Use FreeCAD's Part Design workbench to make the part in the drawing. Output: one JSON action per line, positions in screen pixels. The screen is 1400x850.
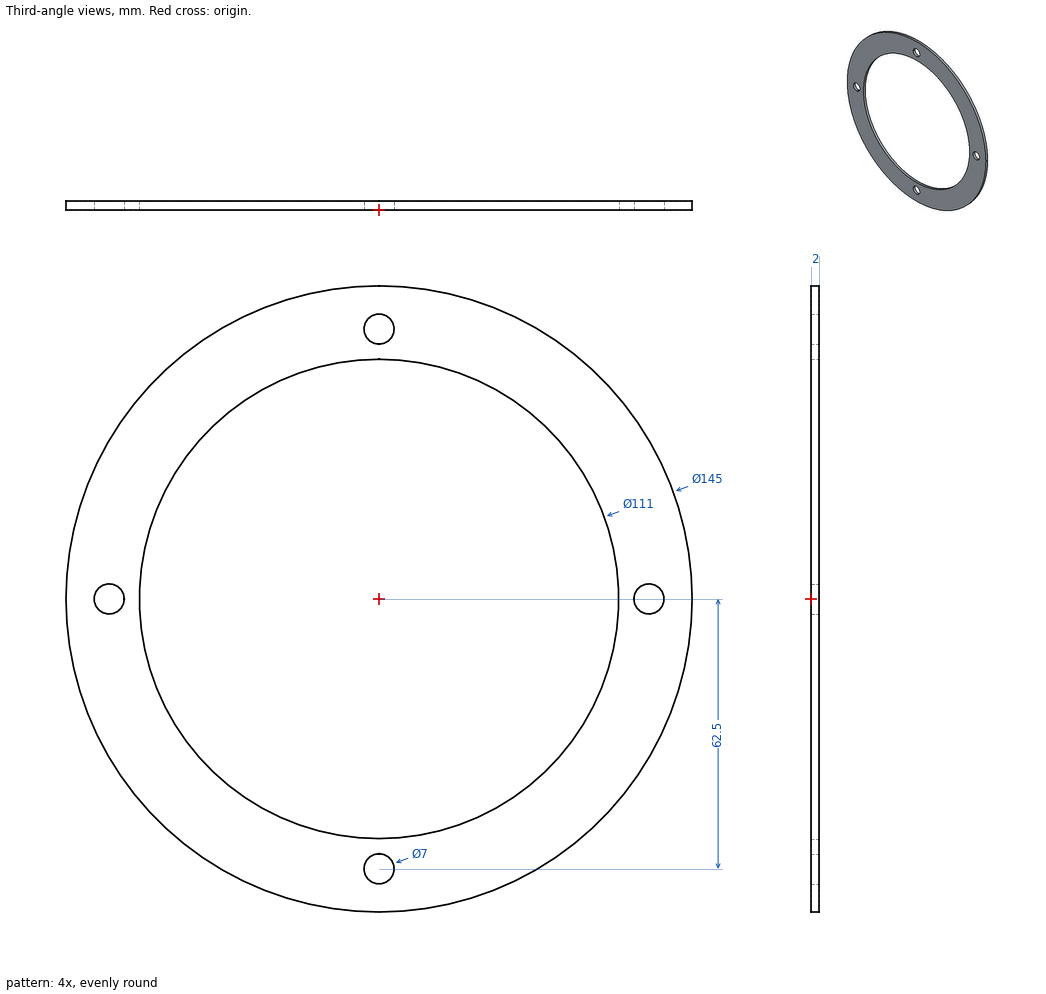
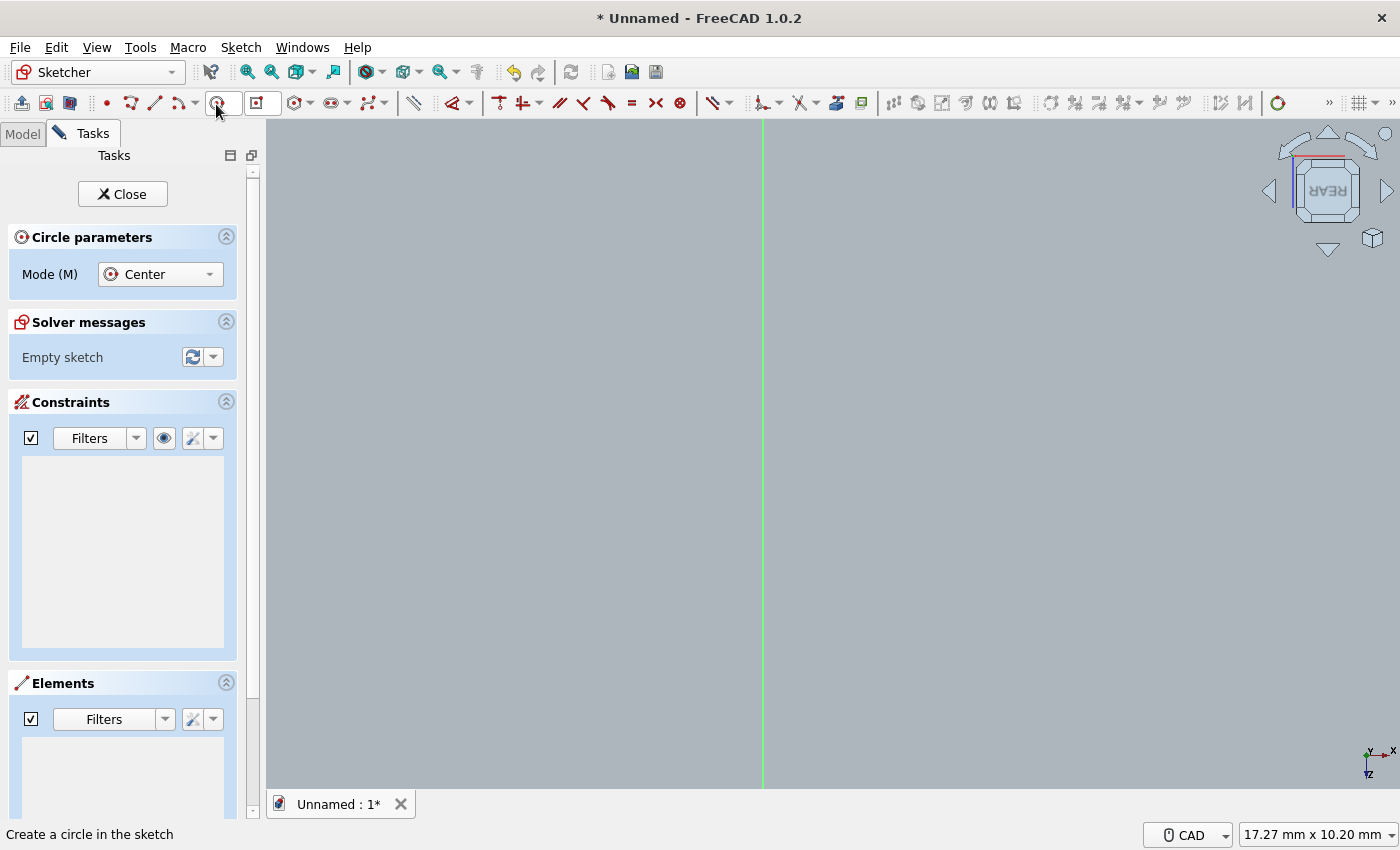
{"action": "left_click", "coordinate": [763, 451]}
{"action": "left_click", "coordinate": [925, 288]}
{"action": "key", "text": "Escape"}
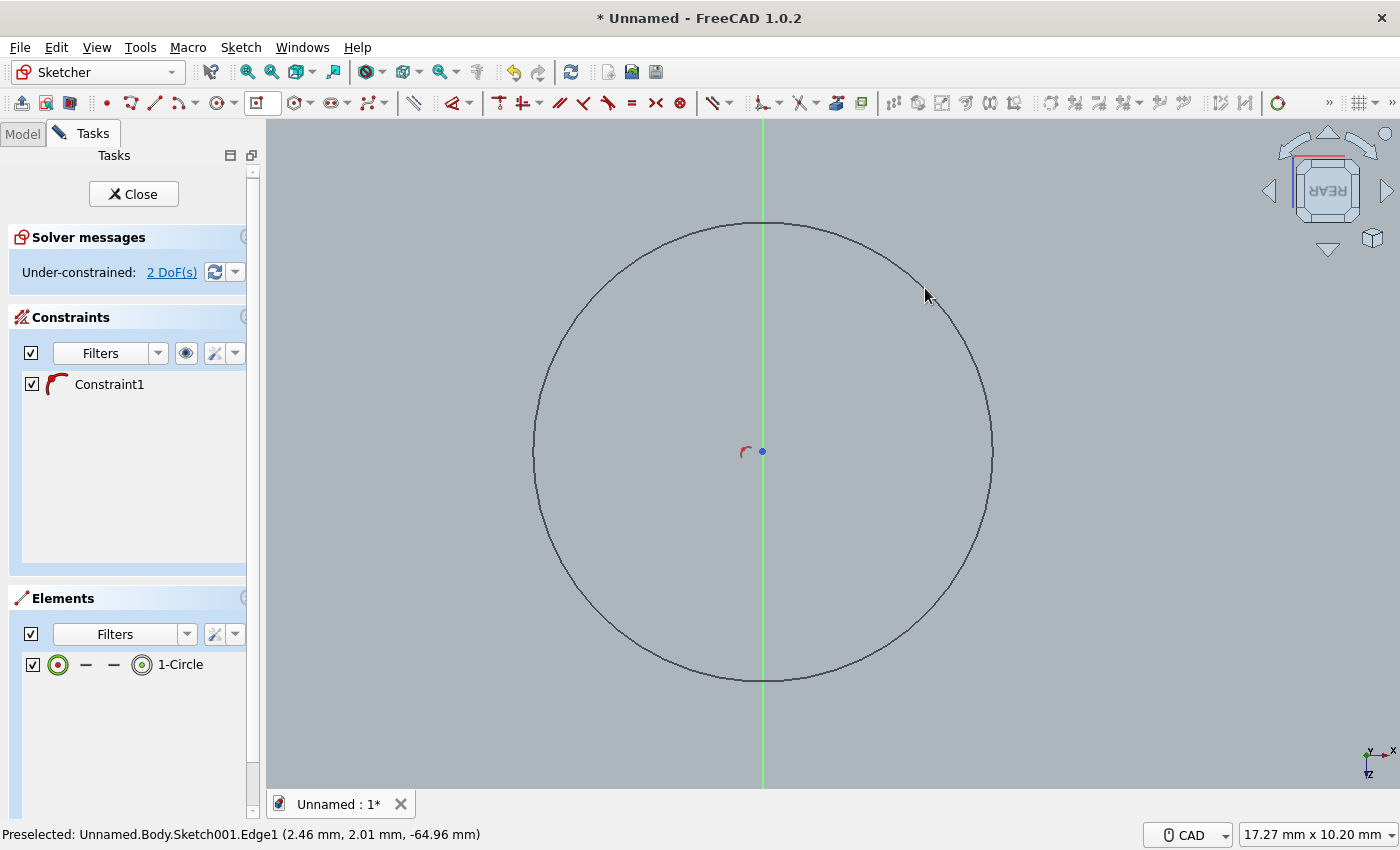
{"action": "left_click", "coordinate": [452, 104]}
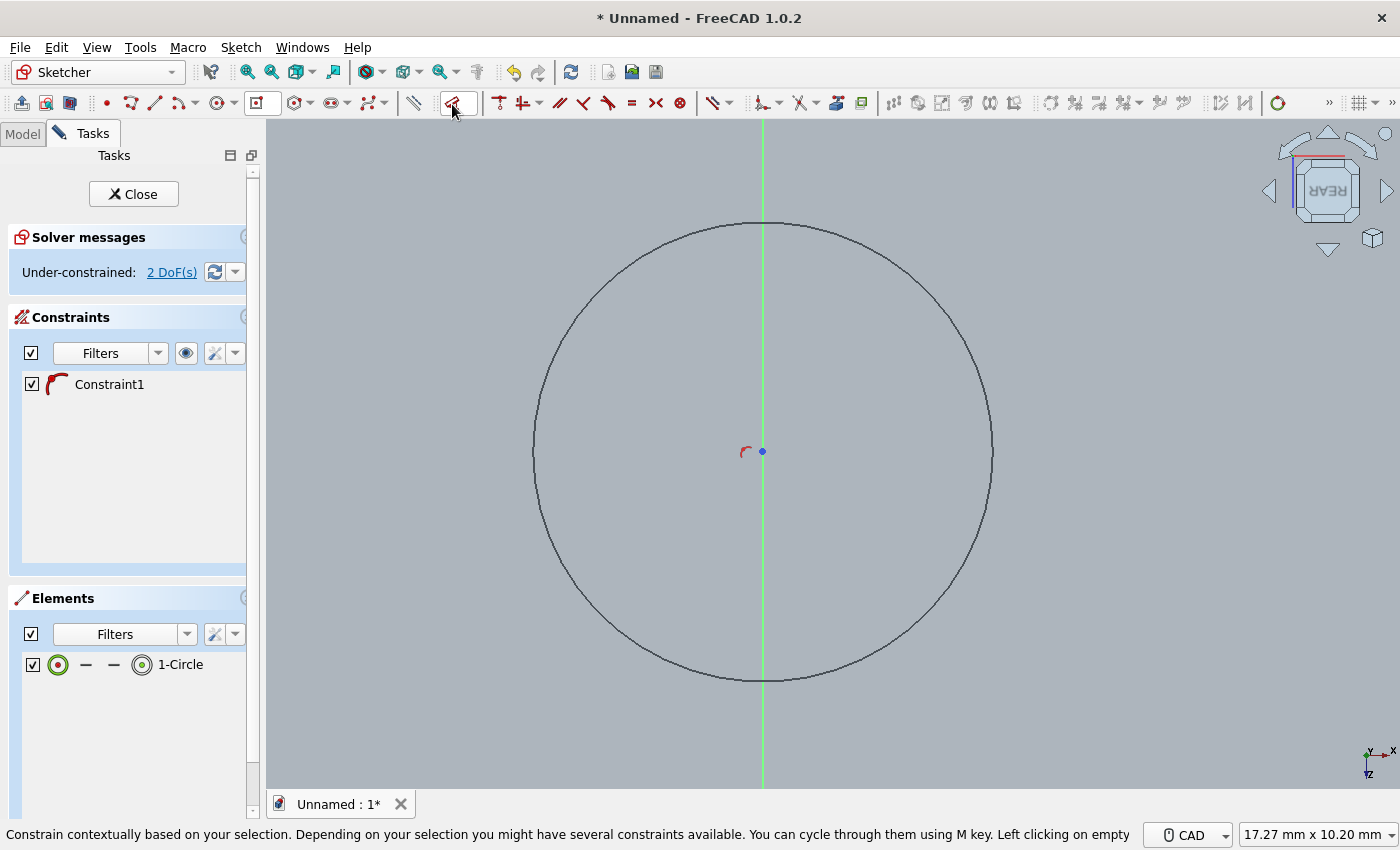
{"action": "left_click", "coordinate": [925, 289]}
{"action": "left_click", "coordinate": [948, 266]}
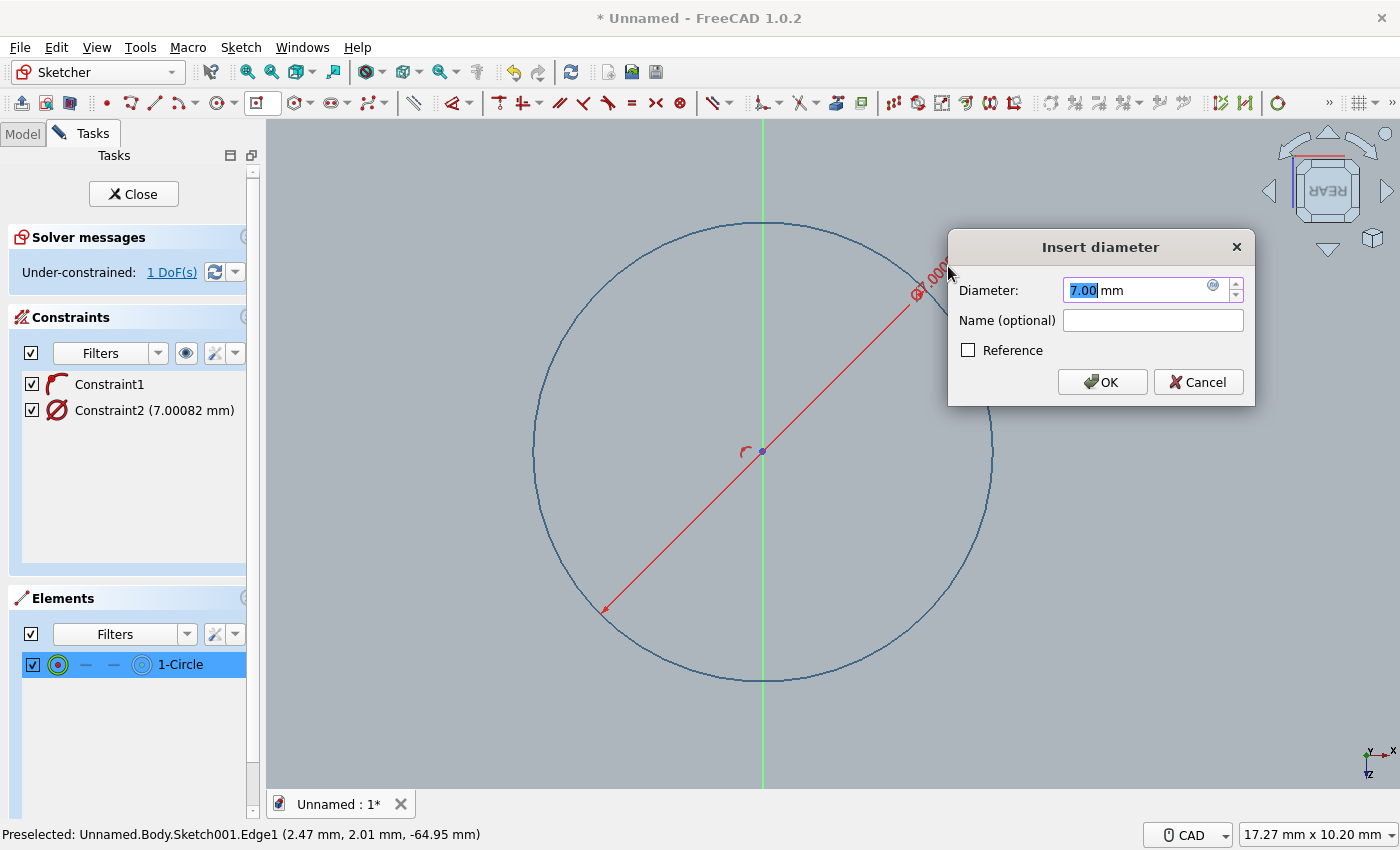
{"action": "type", "text": "7"}
{"action": "key", "text": "Return"}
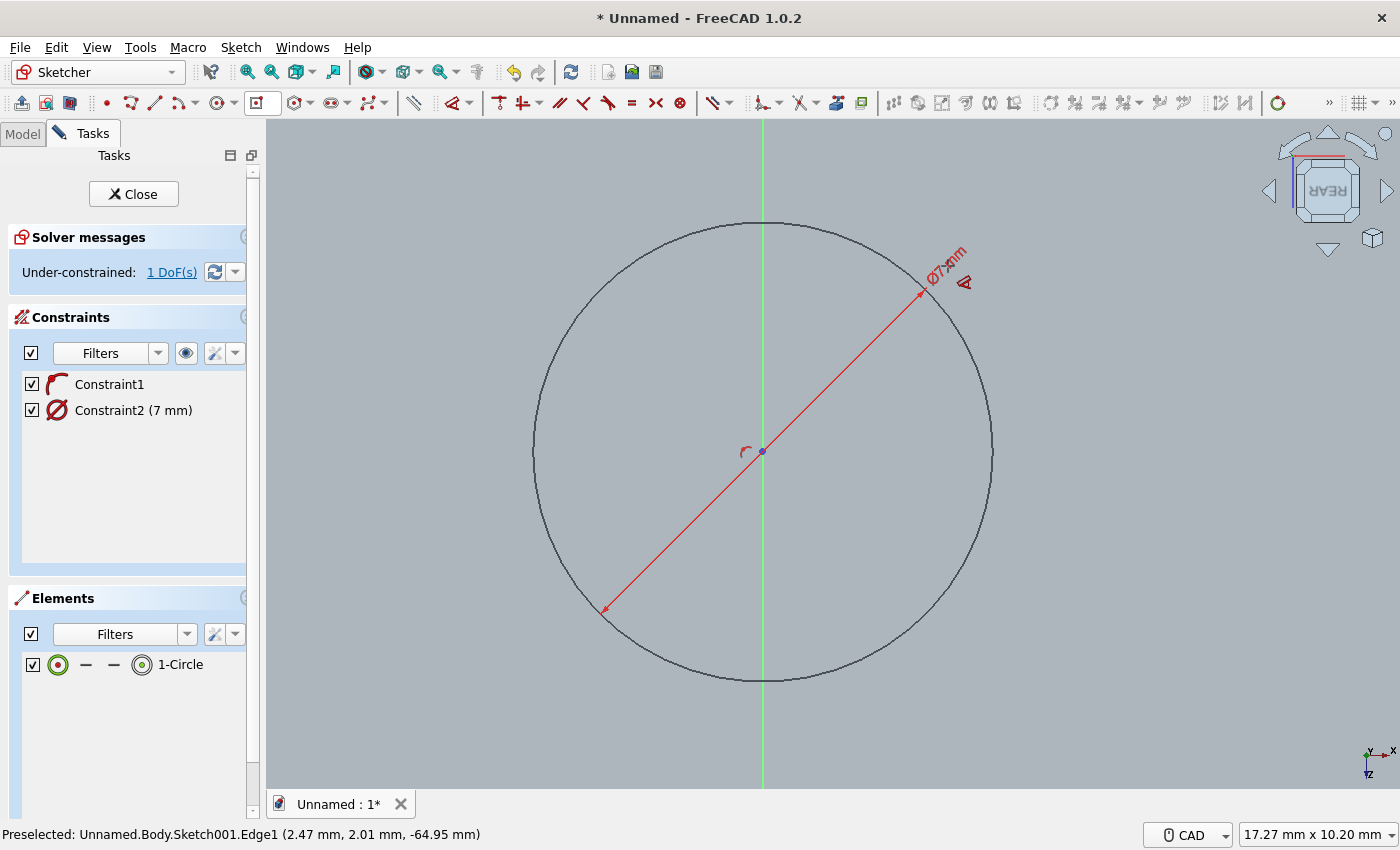
{"action": "left_click", "coordinate": [763, 452]}
{"action": "left_click", "coordinate": [797, 607]}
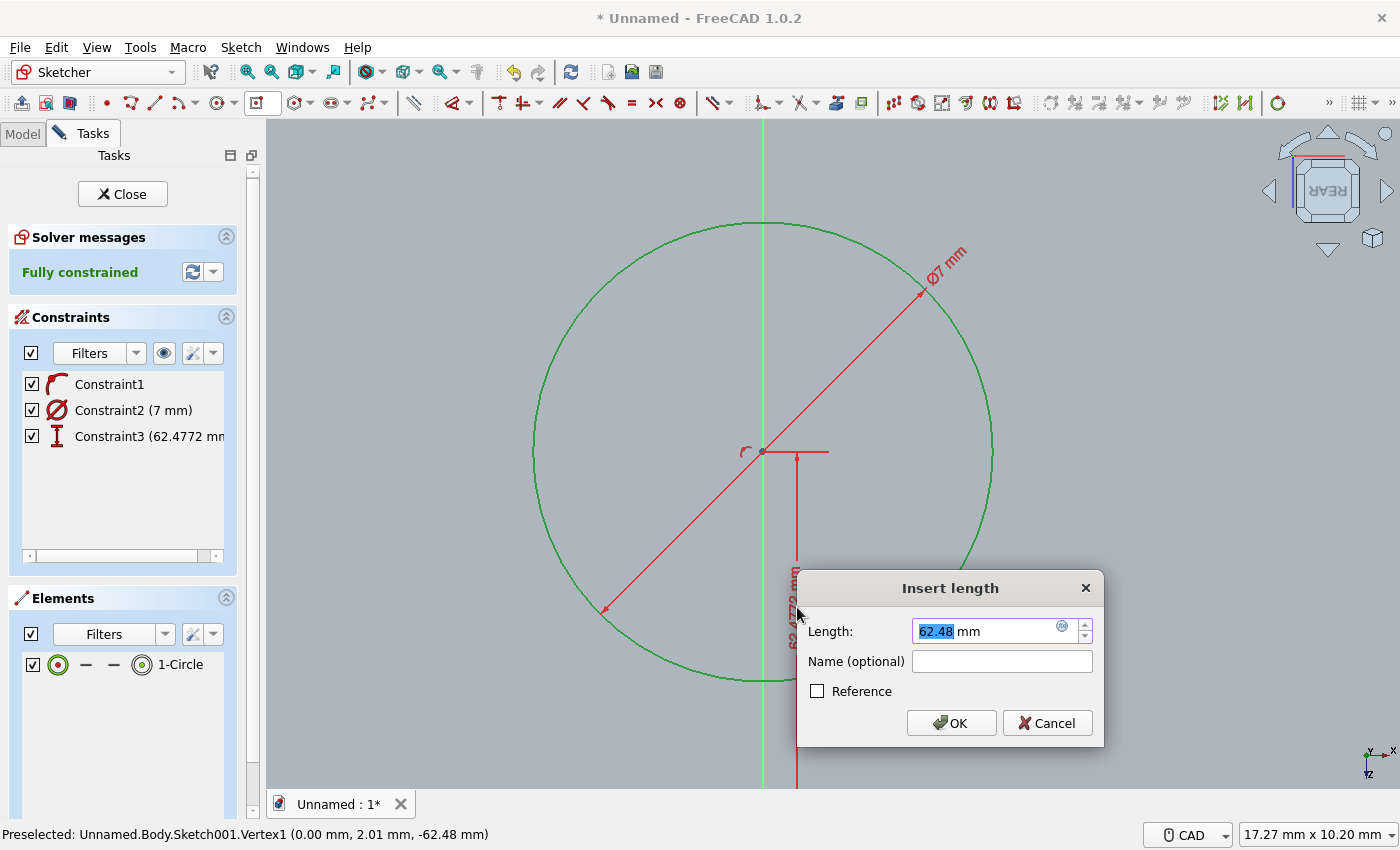
{"action": "type", "text": "62.5"}
{"action": "key", "text": "Return"}
{"action": "key", "text": "Escape"}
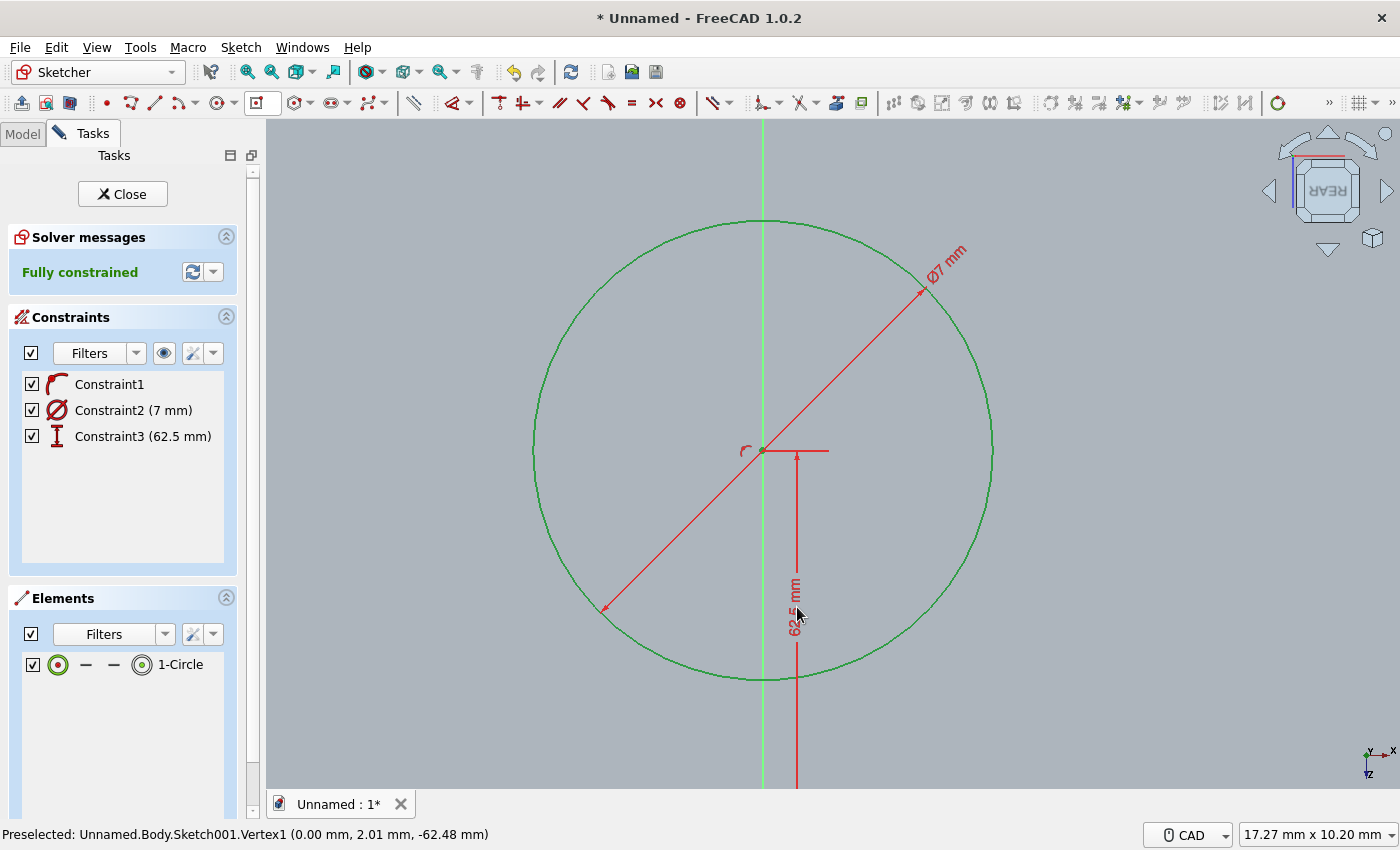
{"action": "left_click", "coordinate": [123, 194]}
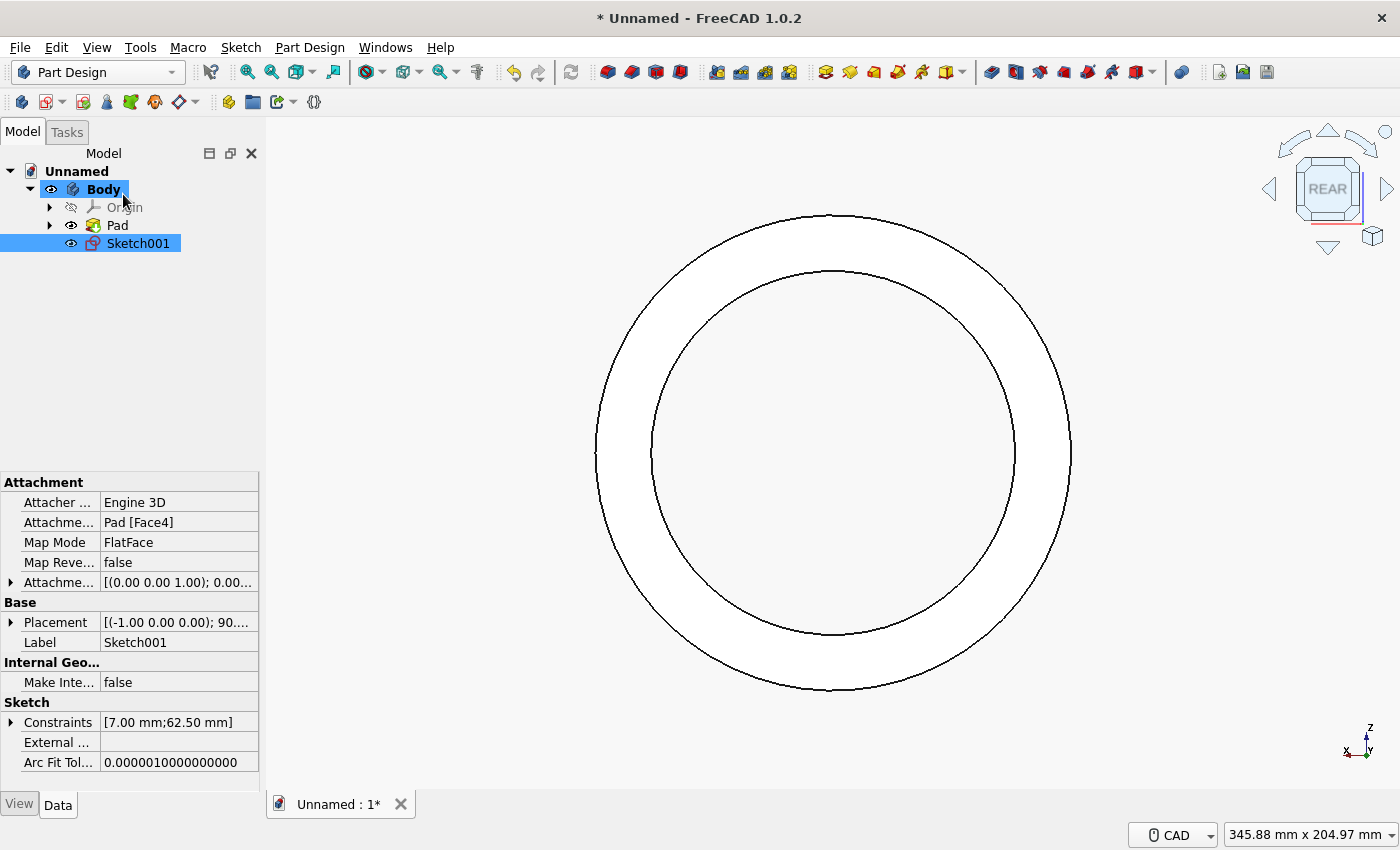
{"action": "left_click", "coordinate": [992, 72]}